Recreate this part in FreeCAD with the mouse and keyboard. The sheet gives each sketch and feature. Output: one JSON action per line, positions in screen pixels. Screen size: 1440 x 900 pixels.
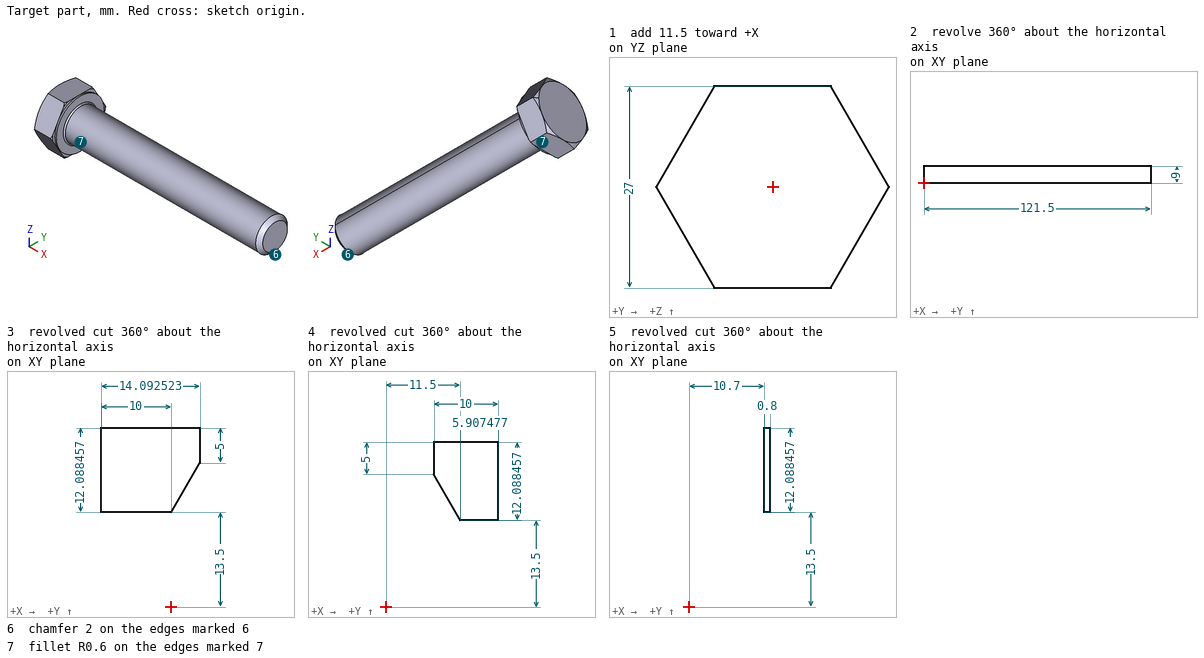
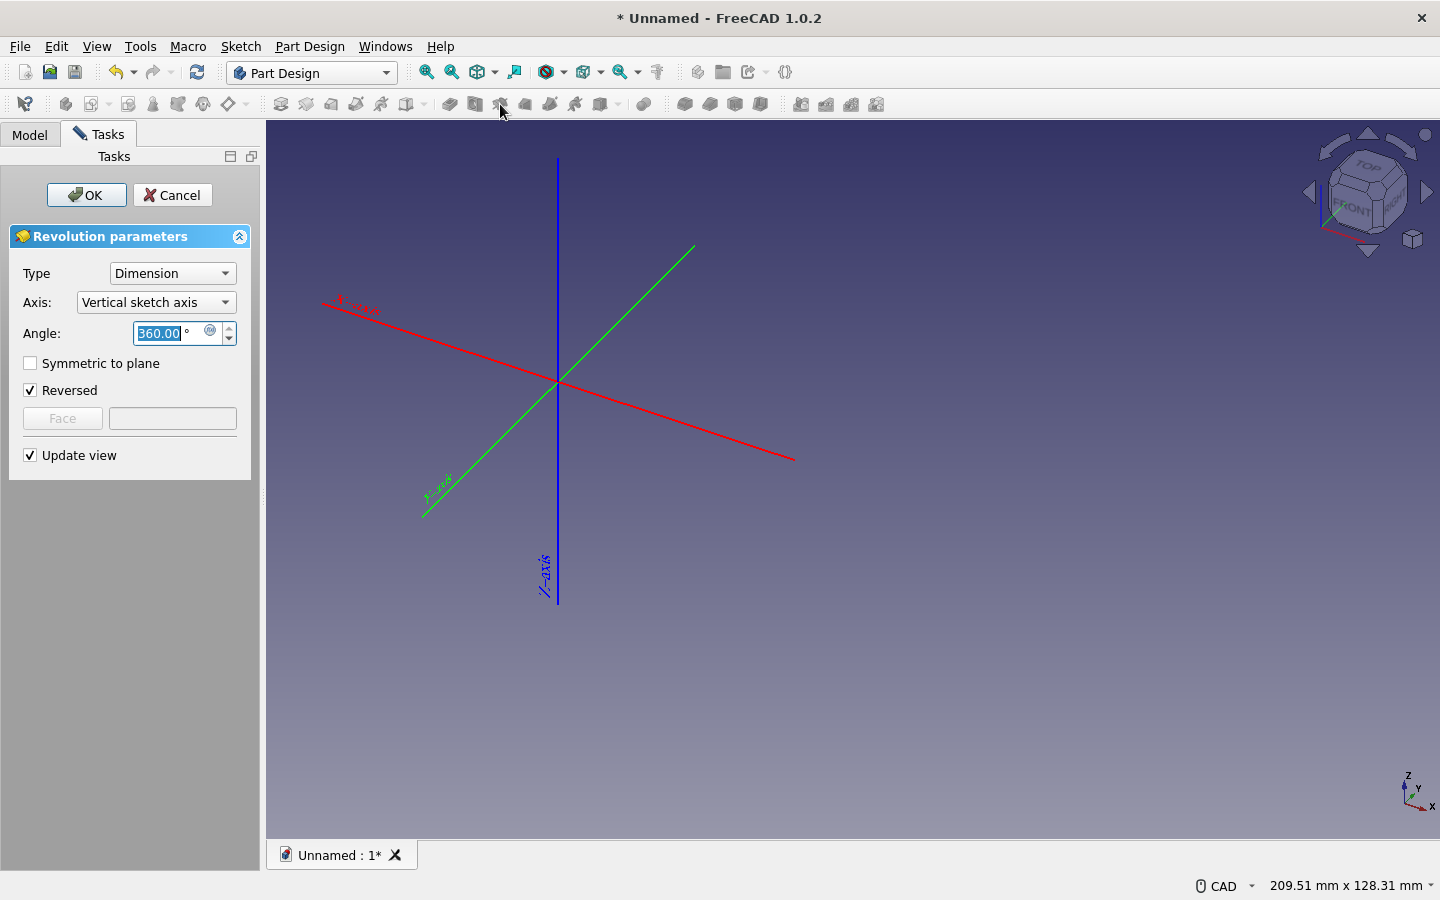
{"action": "left_click", "coordinate": [157, 302]}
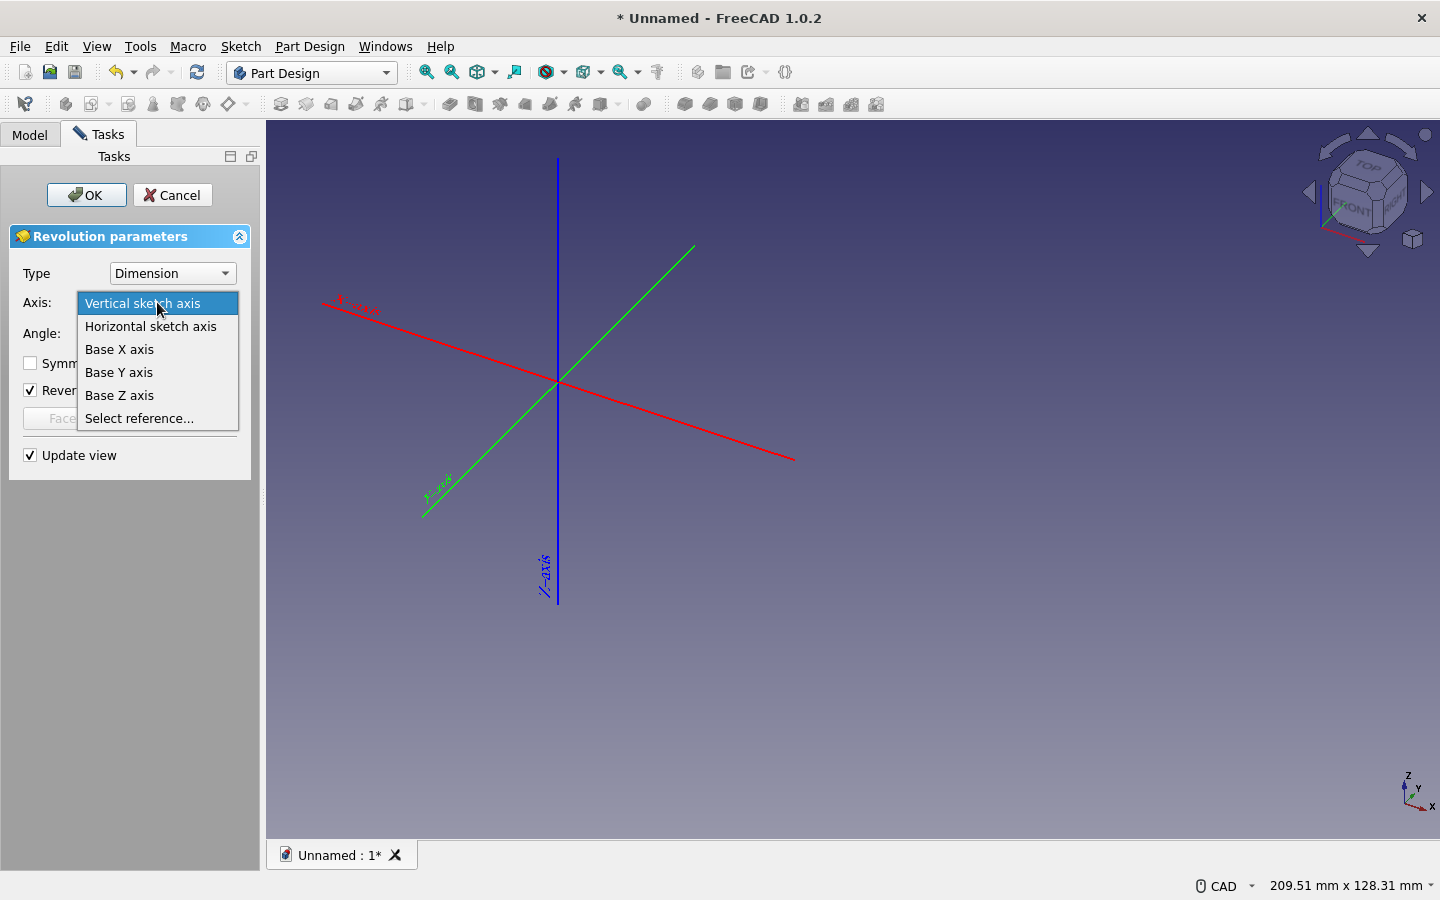
{"action": "left_click", "coordinate": [156, 326]}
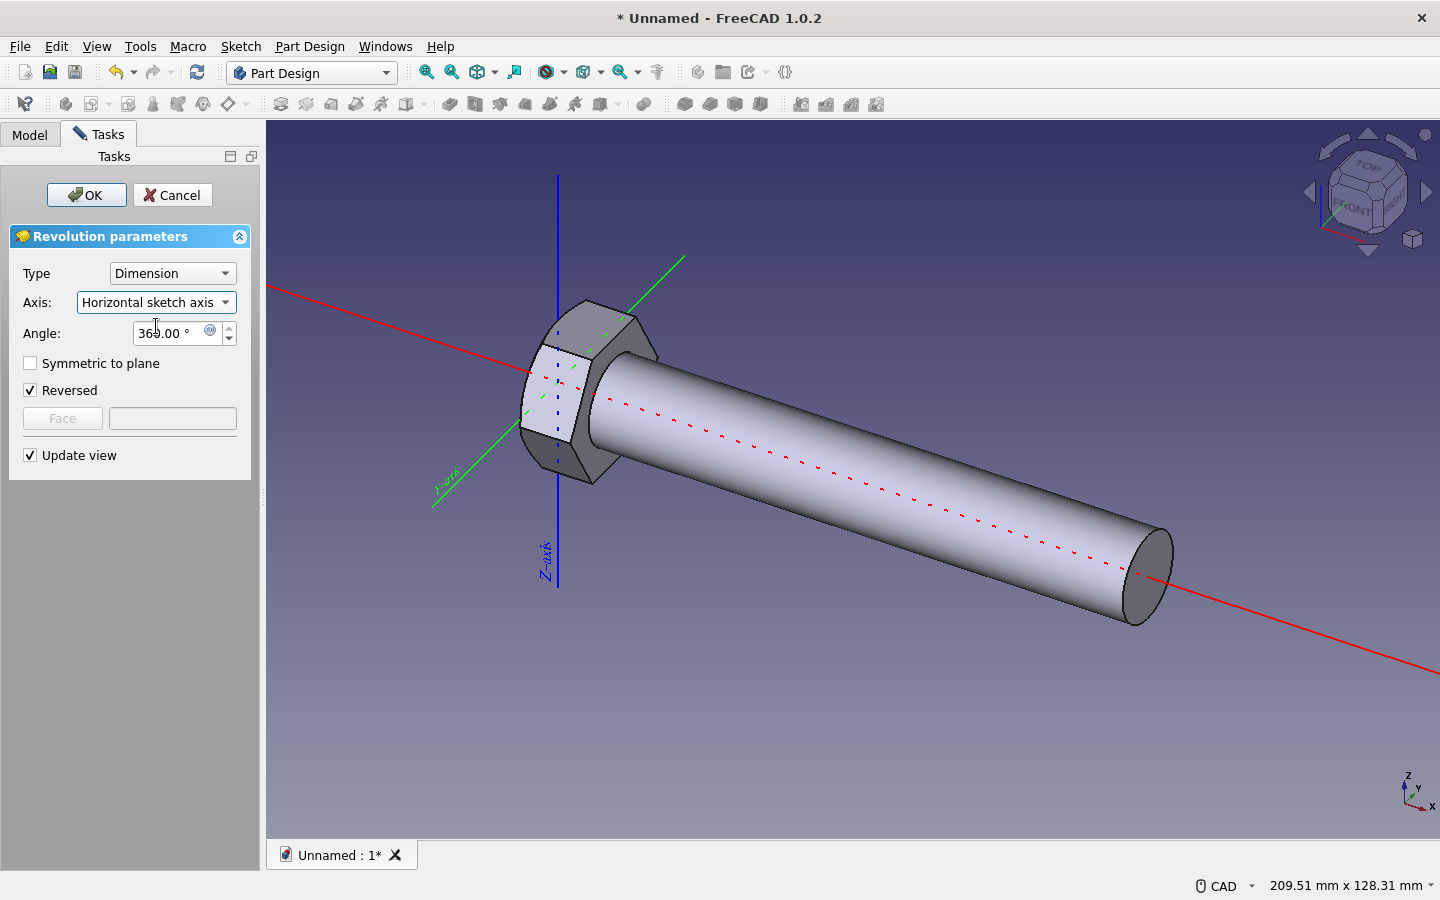
{"action": "left_click", "coordinate": [87, 195]}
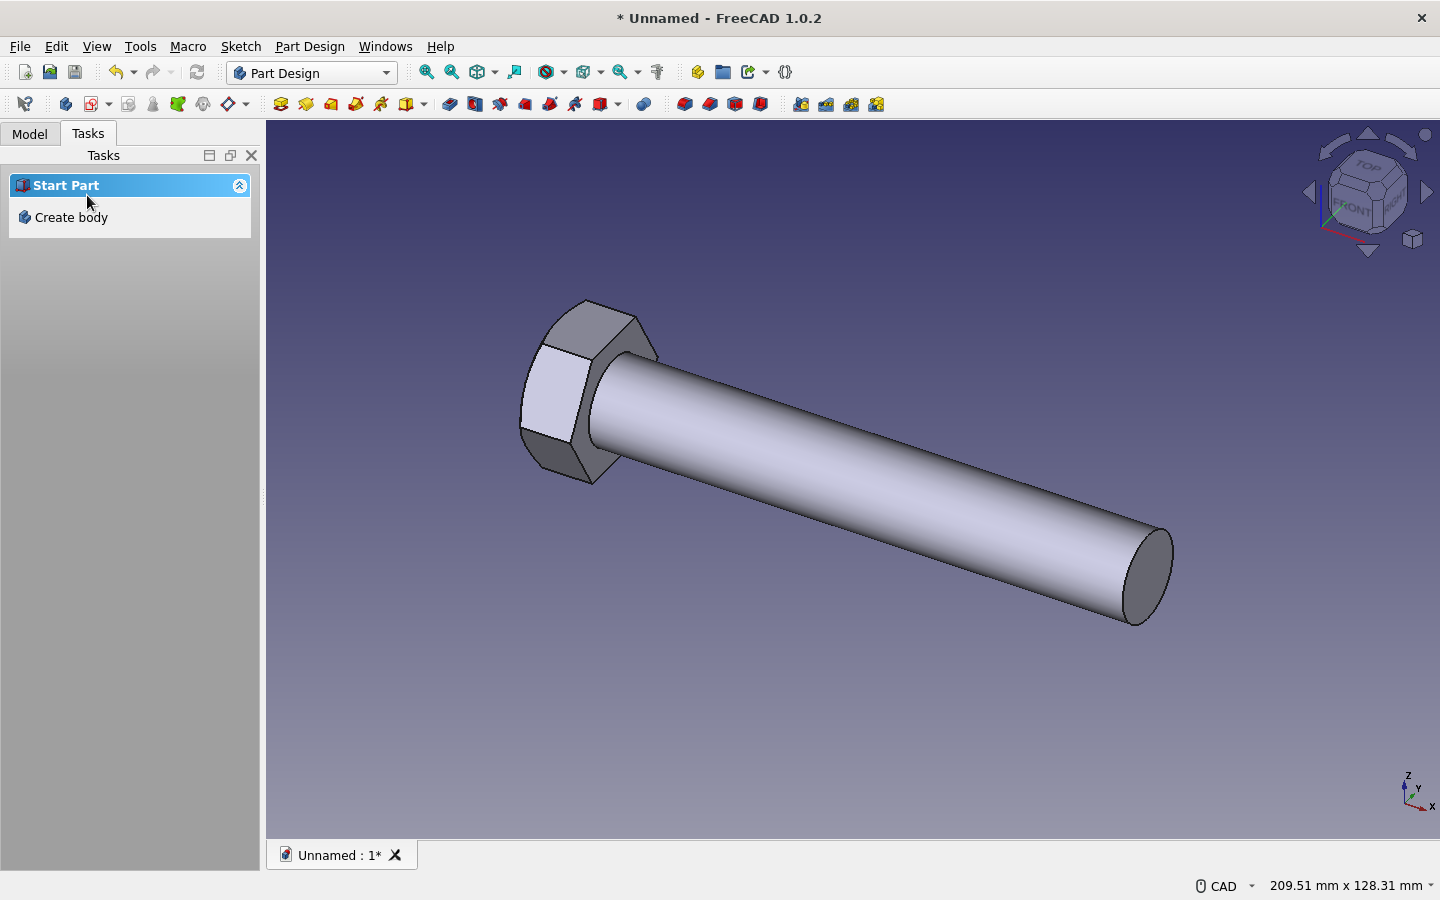
{"action": "left_click", "coordinate": [90, 104]}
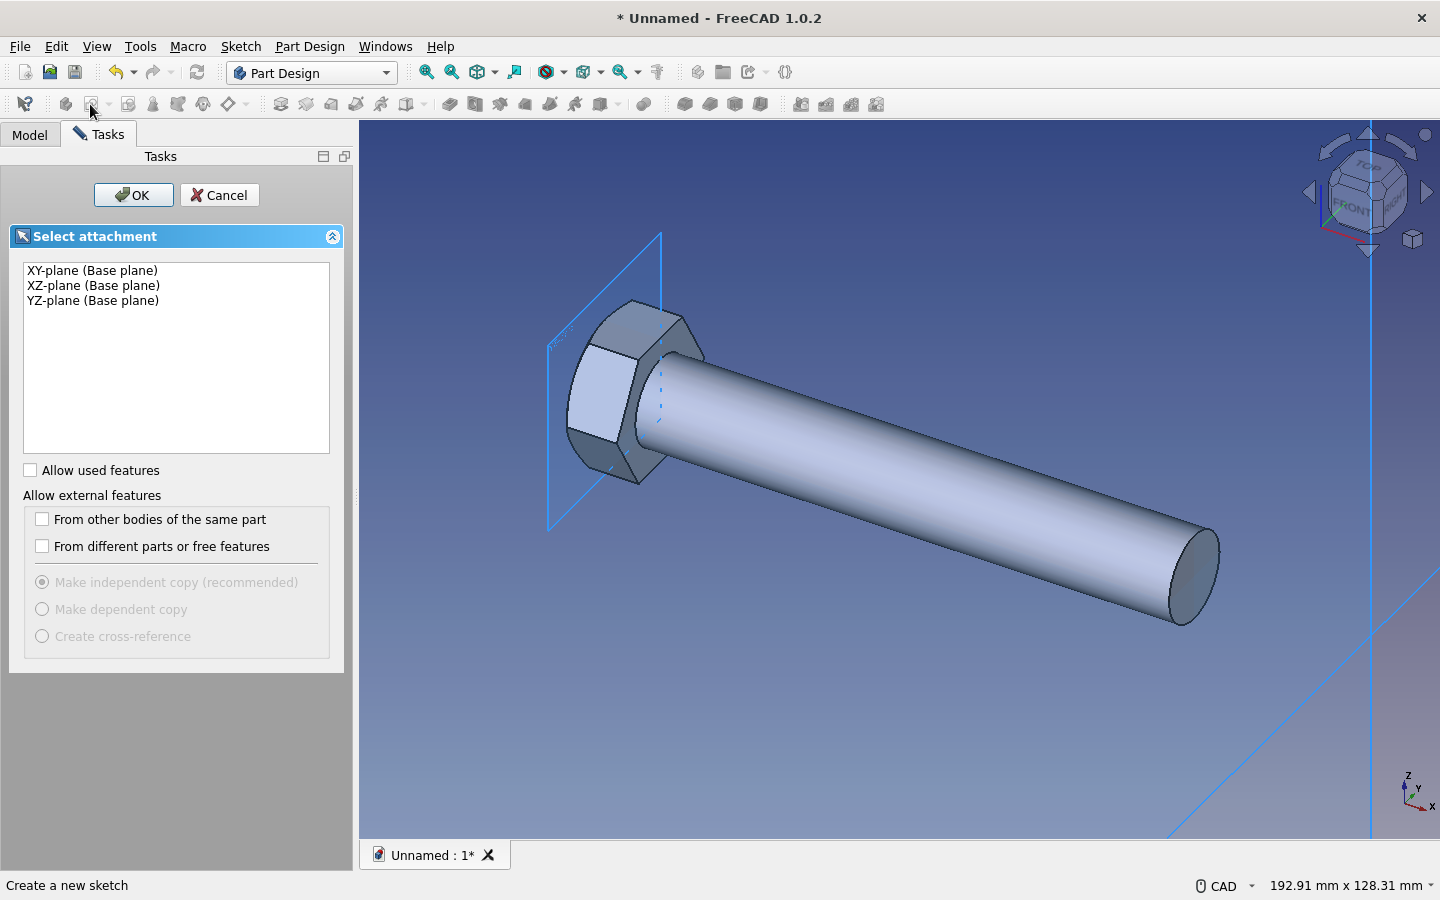
{"action": "left_click", "coordinate": [84, 270]}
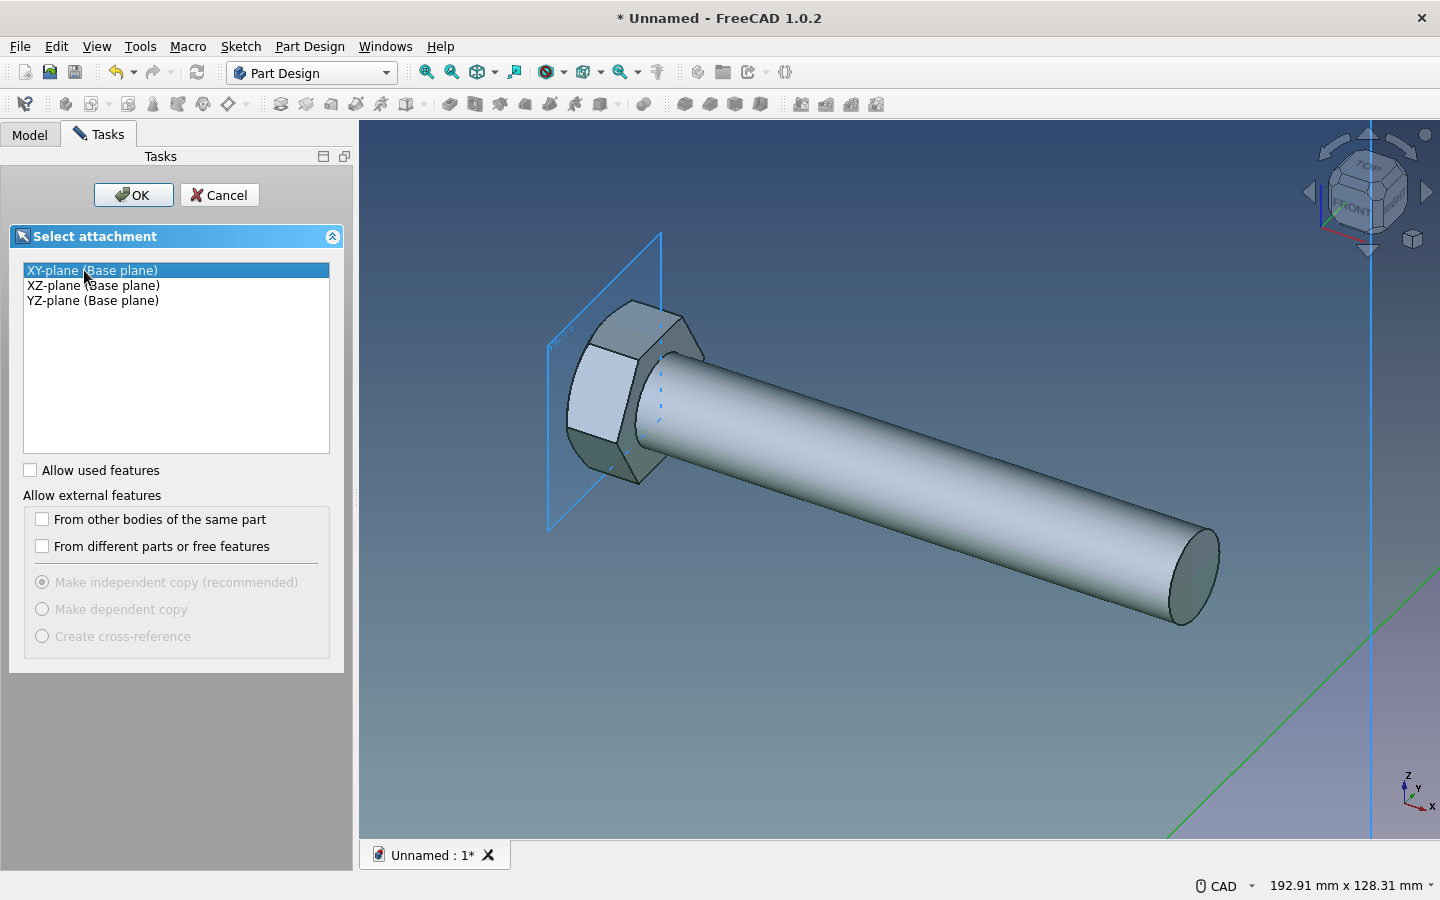
{"action": "left_click", "coordinate": [134, 195]}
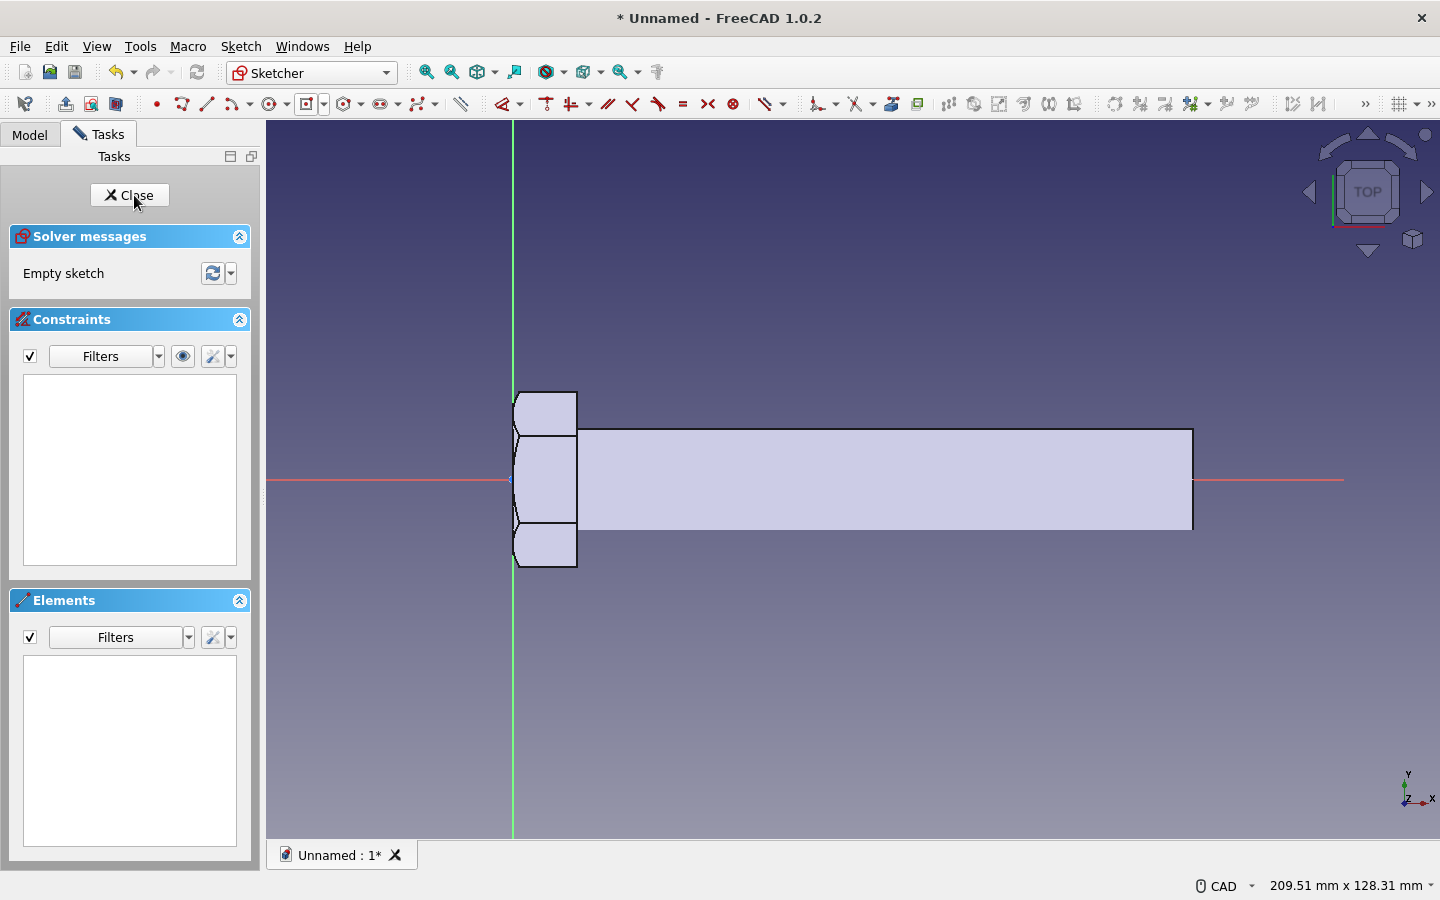
{"action": "left_click", "coordinate": [116, 104]}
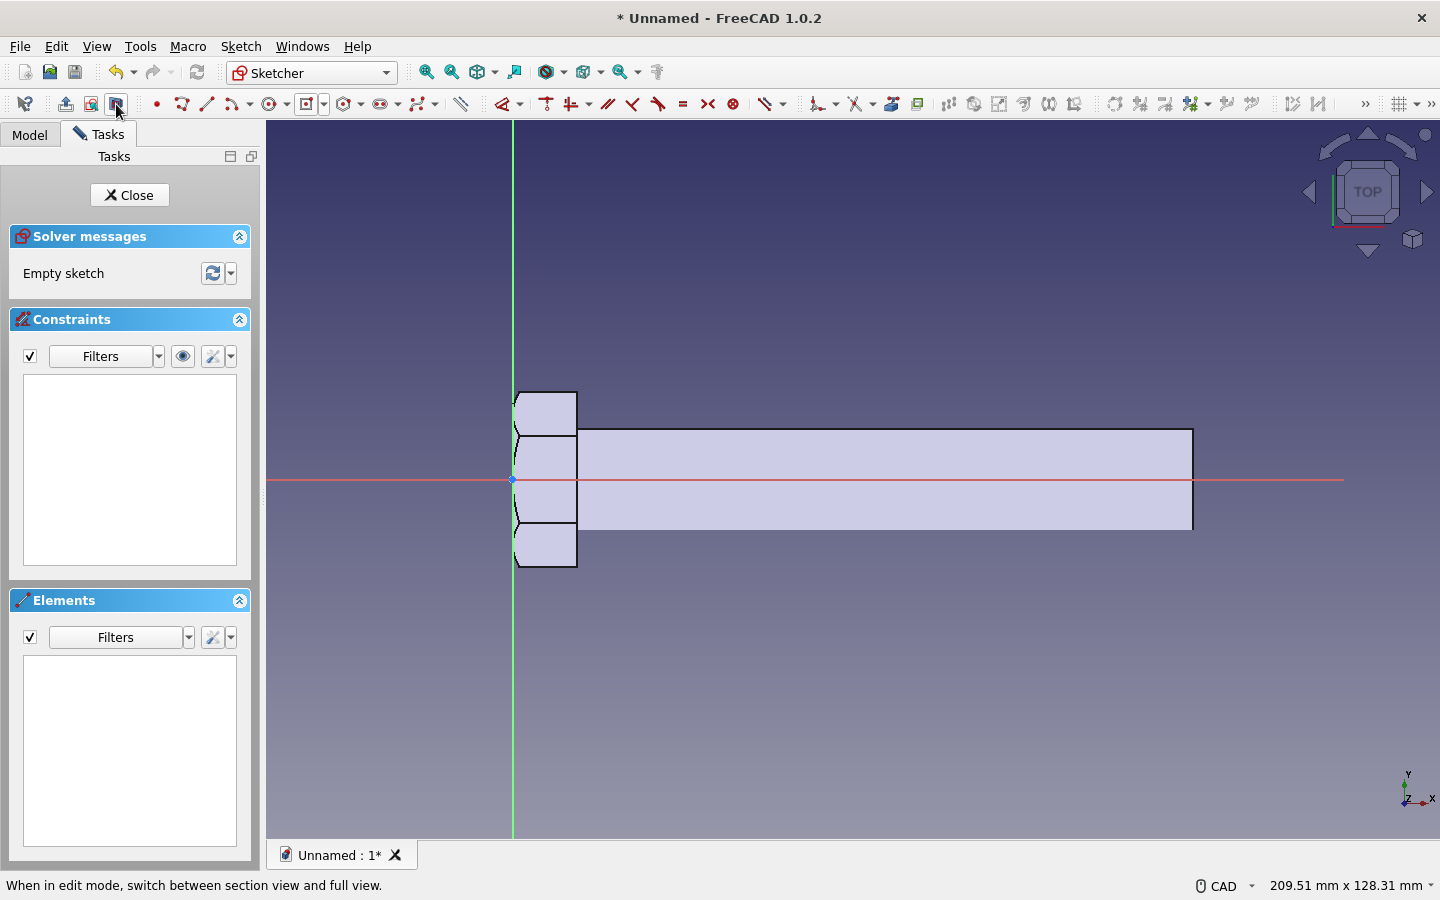
{"action": "scroll", "coordinate": [465, 377], "scroll_direction": "up", "scroll_amount": 6}